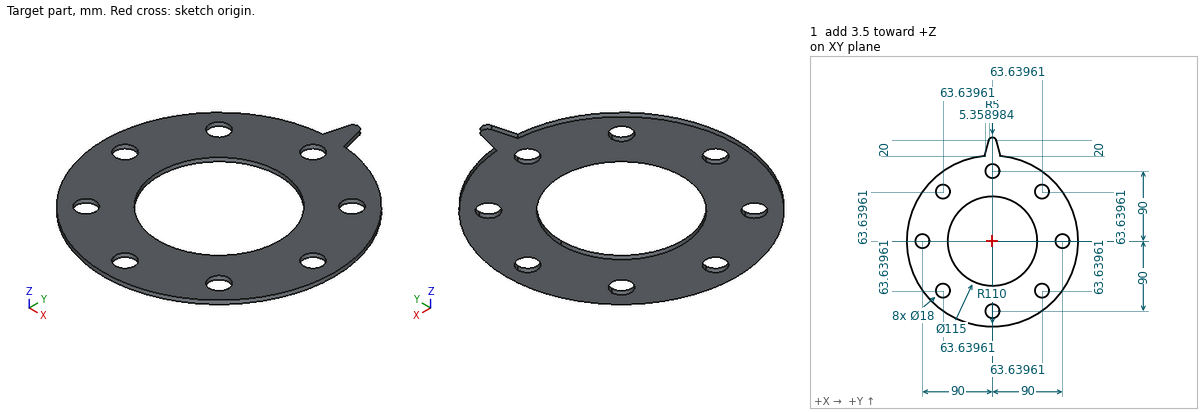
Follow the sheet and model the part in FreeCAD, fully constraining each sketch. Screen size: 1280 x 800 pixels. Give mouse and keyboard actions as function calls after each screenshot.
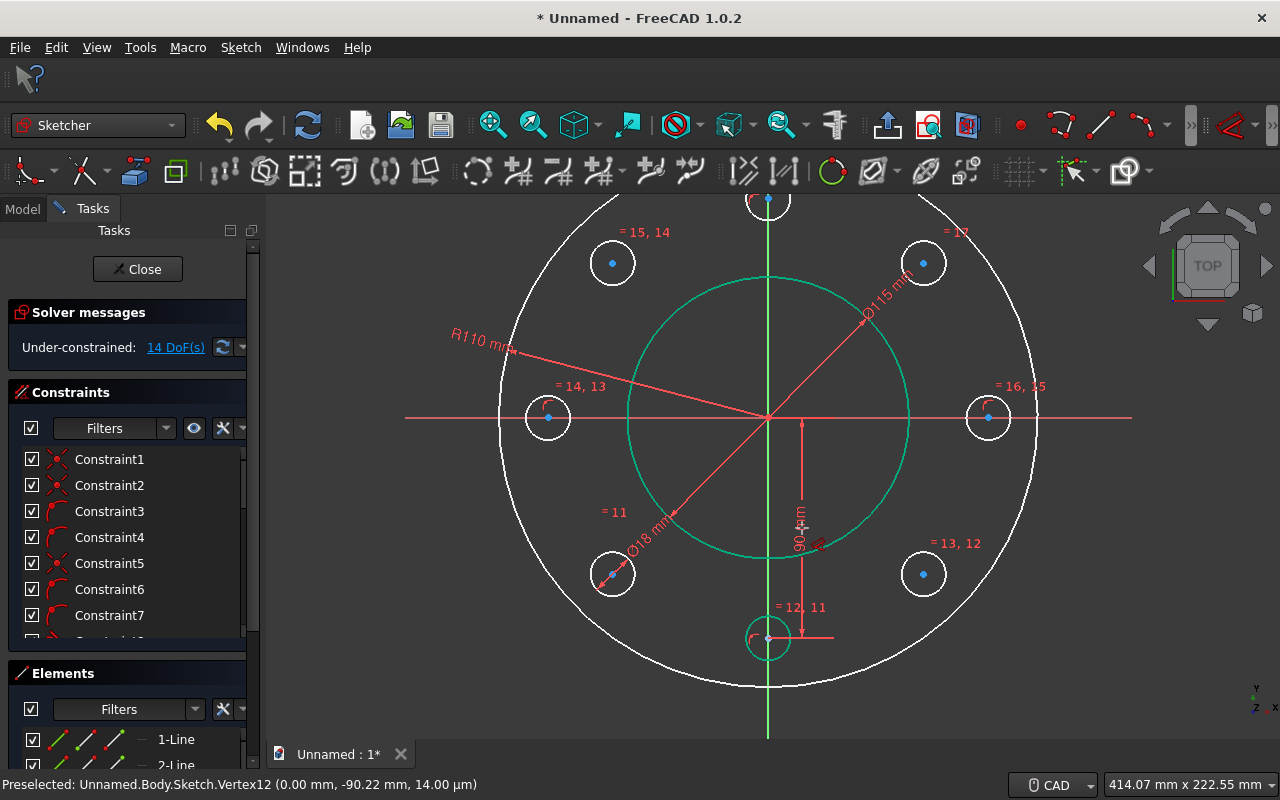
click(548, 418)
click(658, 452)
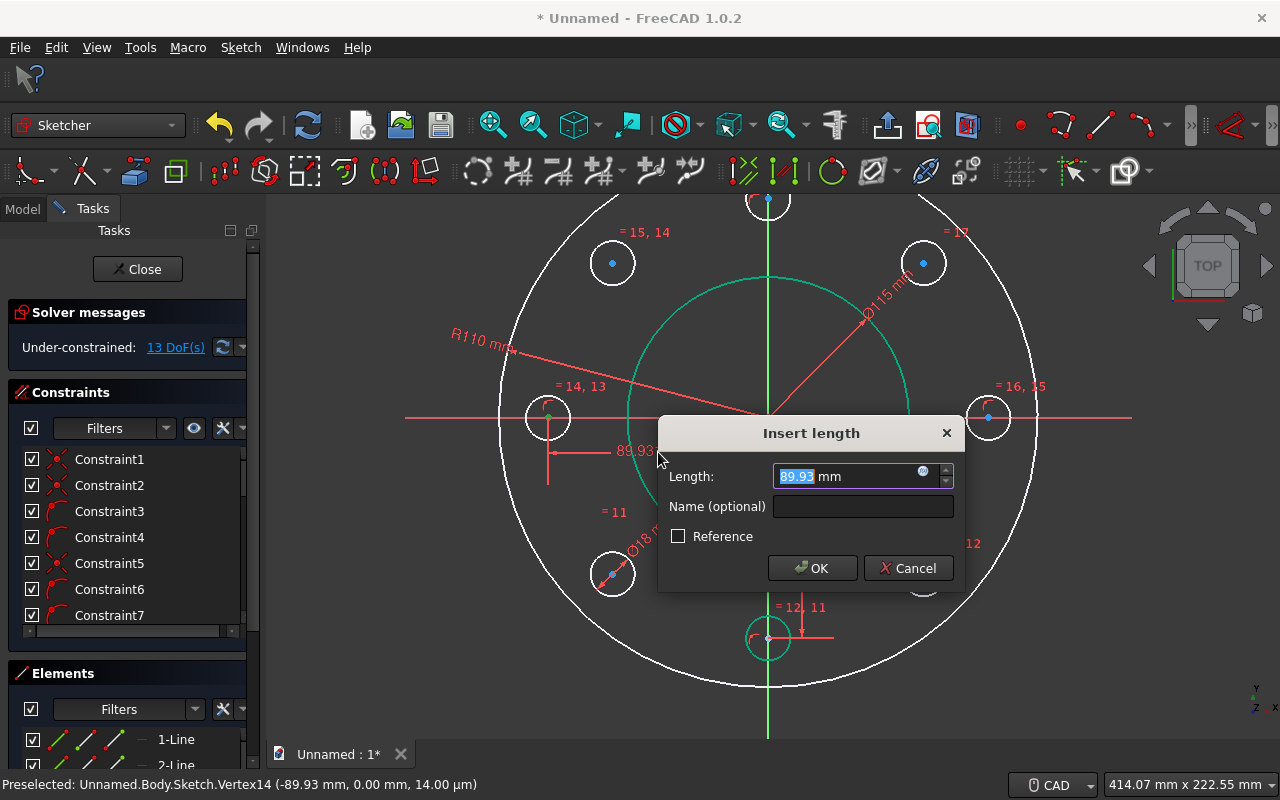
text(90)
key(Return)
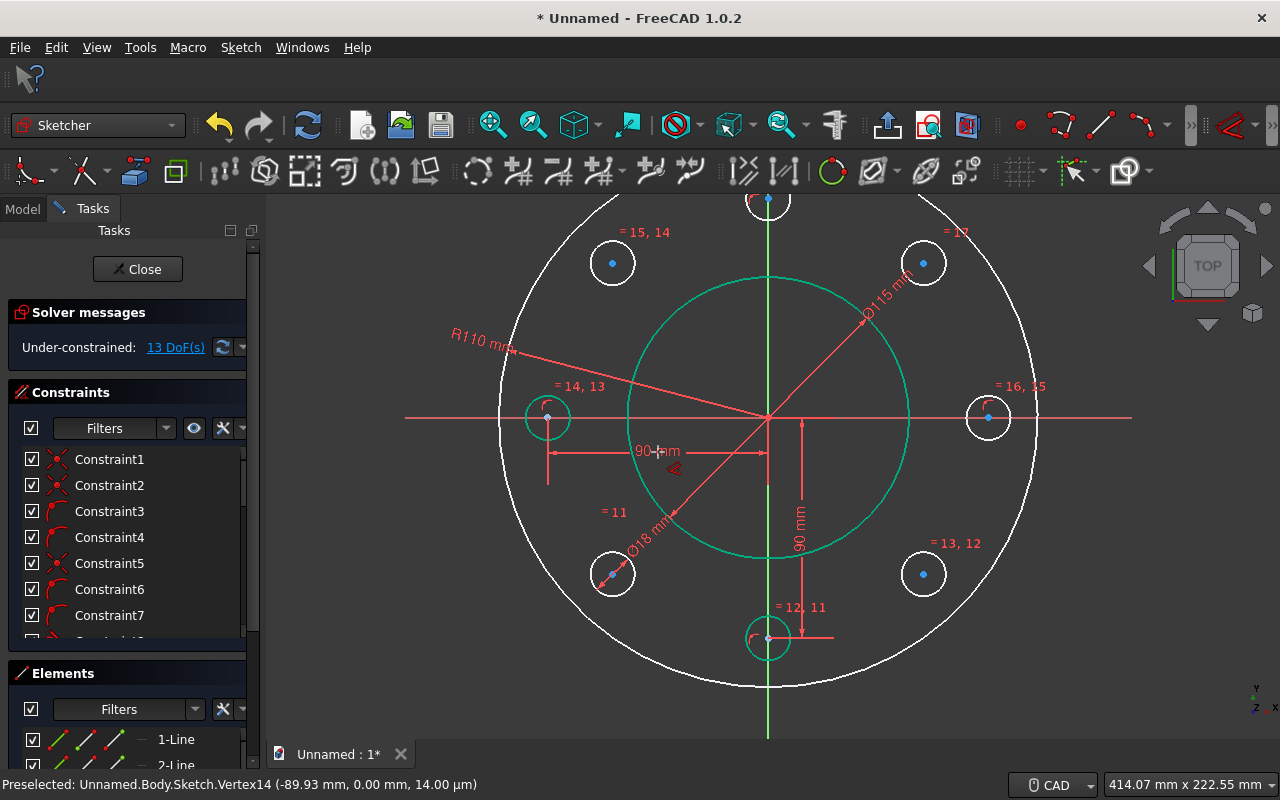
click(988, 418)
click(878, 452)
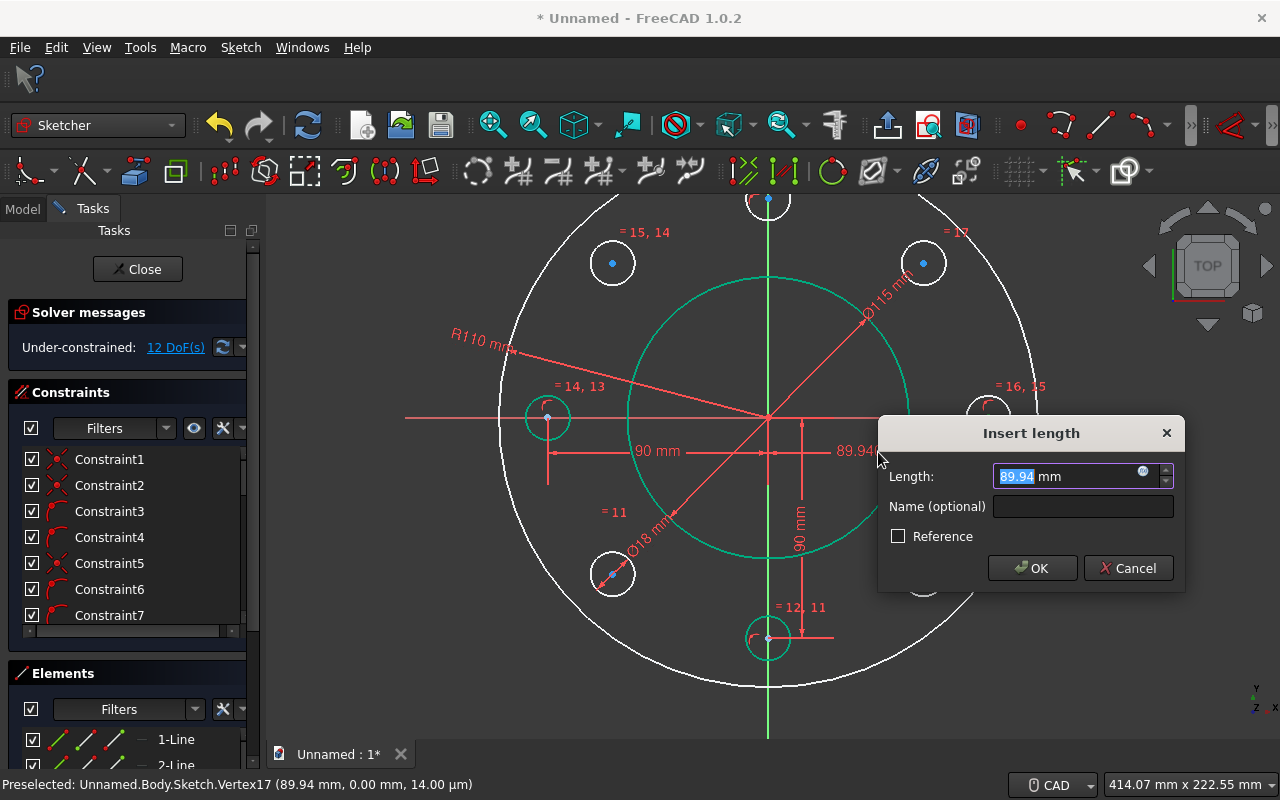
text(90)
key(Return)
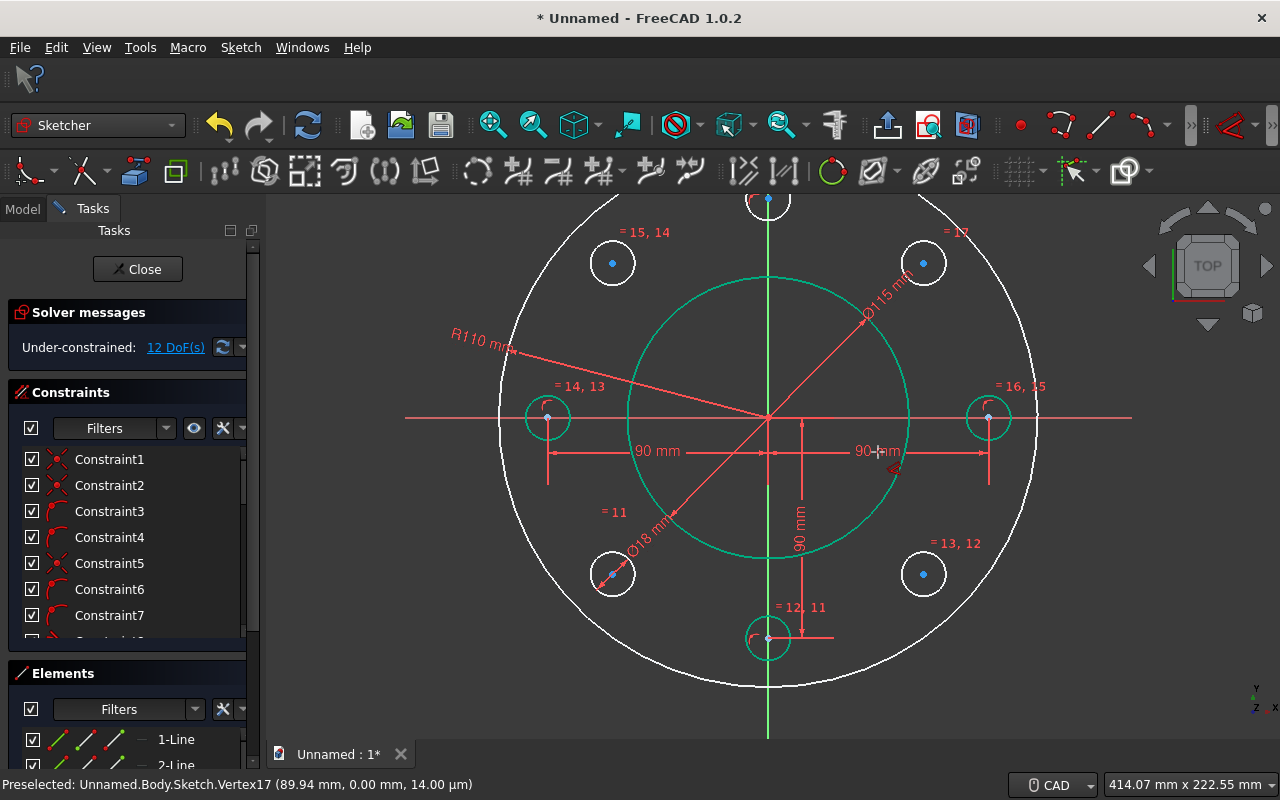
scroll(627, 560, down, 3)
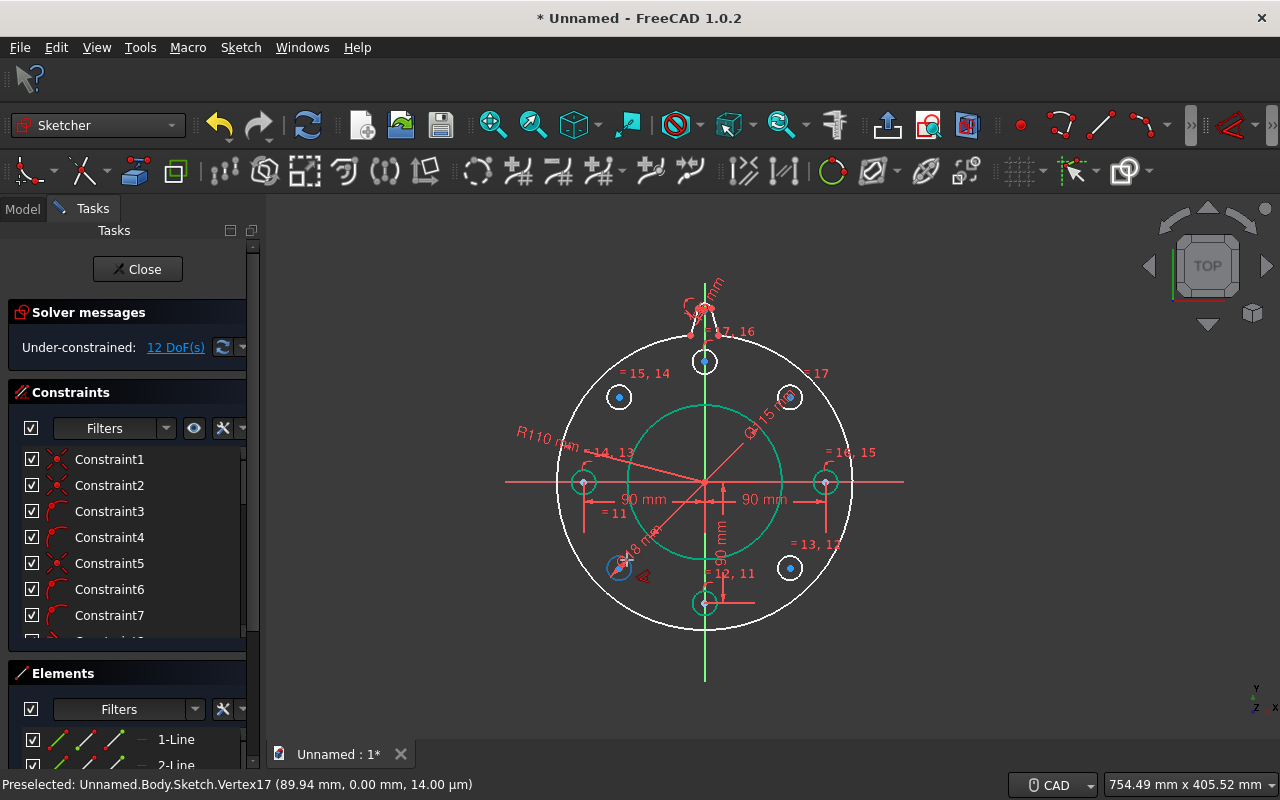
click(705, 362)
click(739, 394)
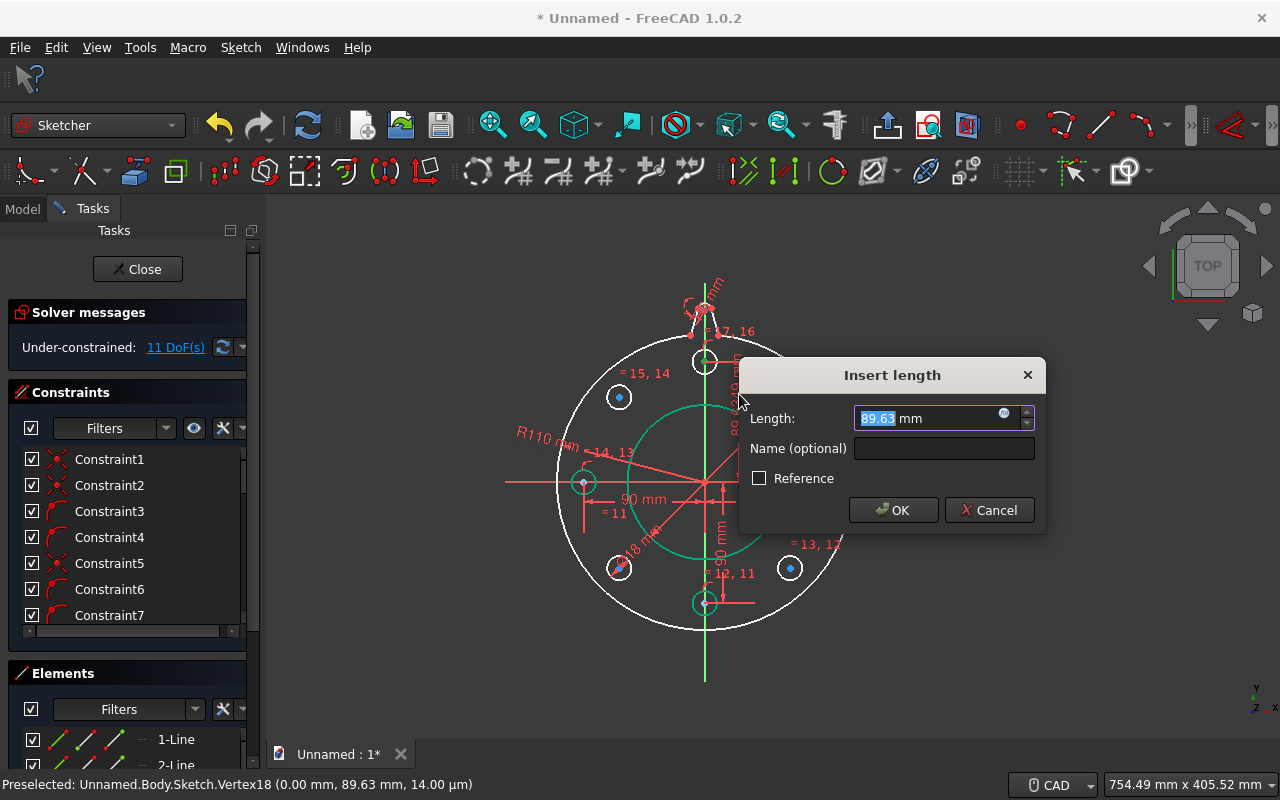
text(90)
key(Return)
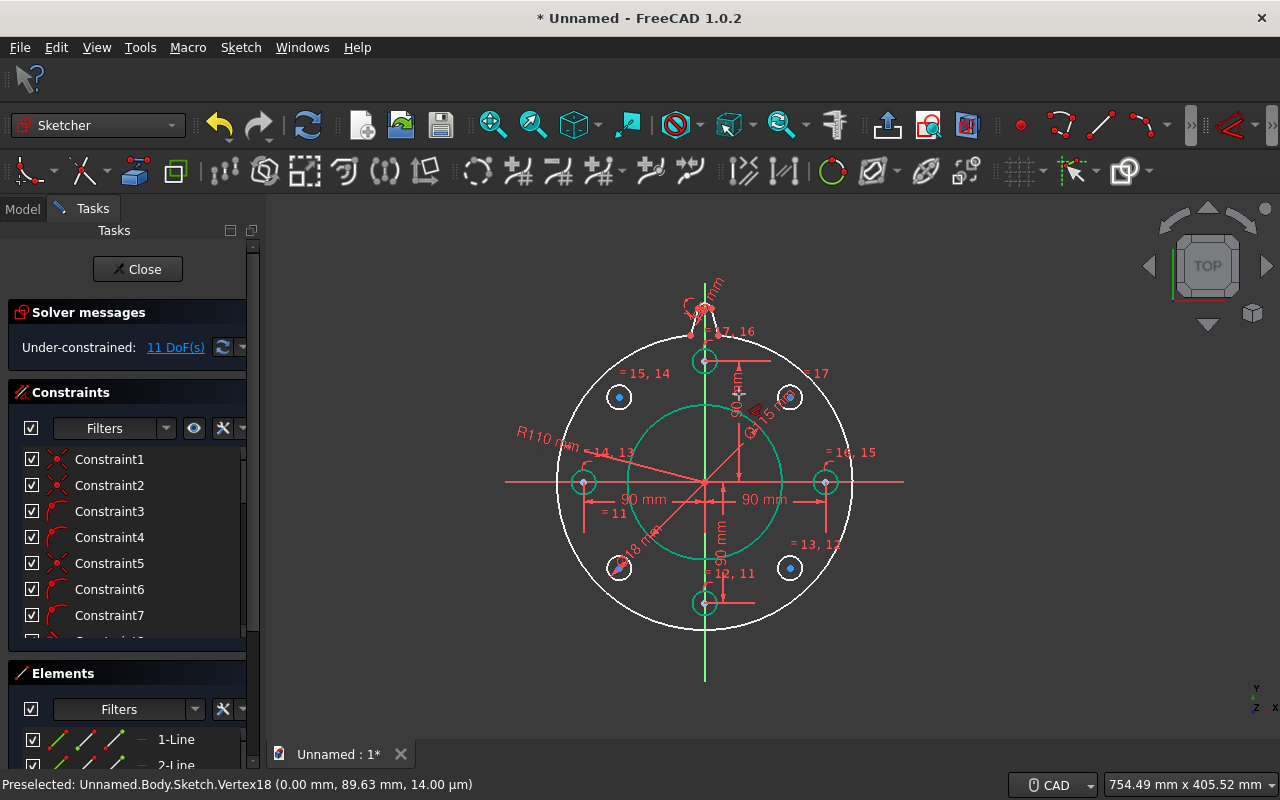
scroll(695, 319, up, 2)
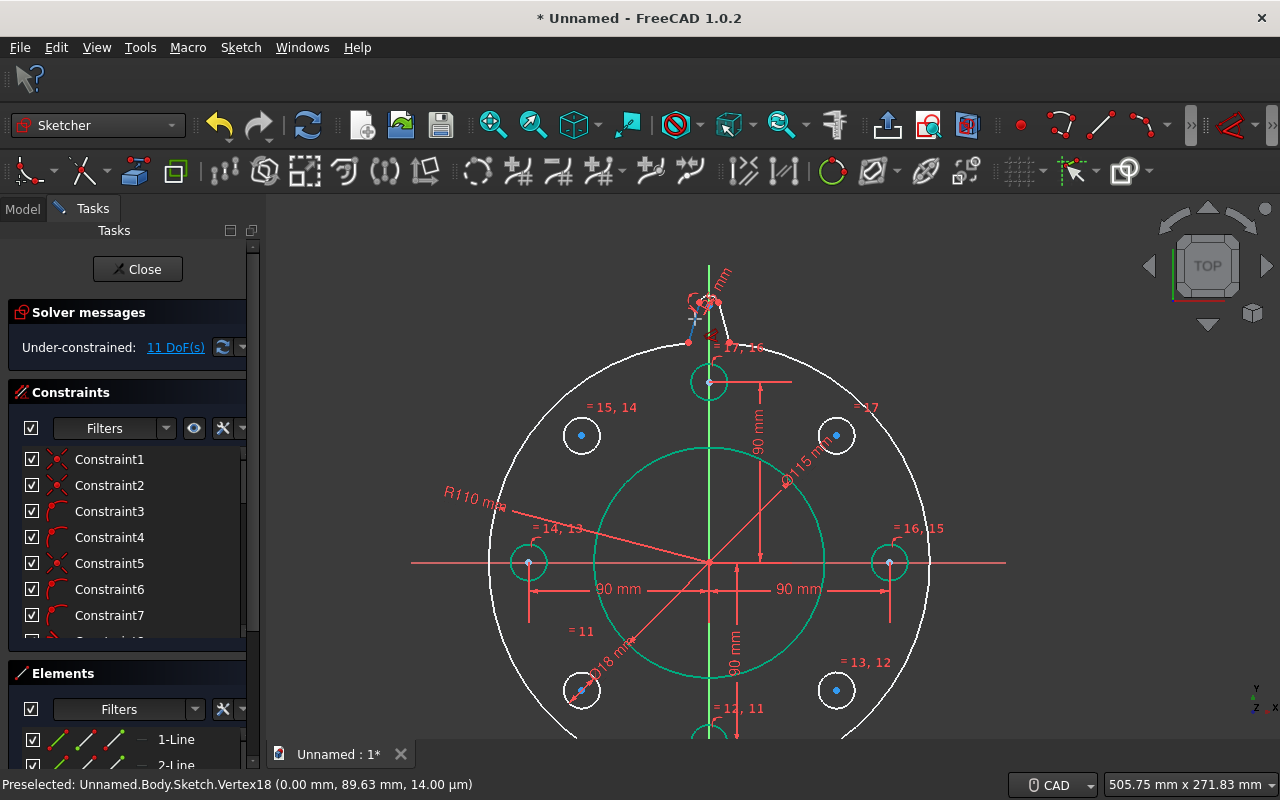
click(695, 319)
click(655, 323)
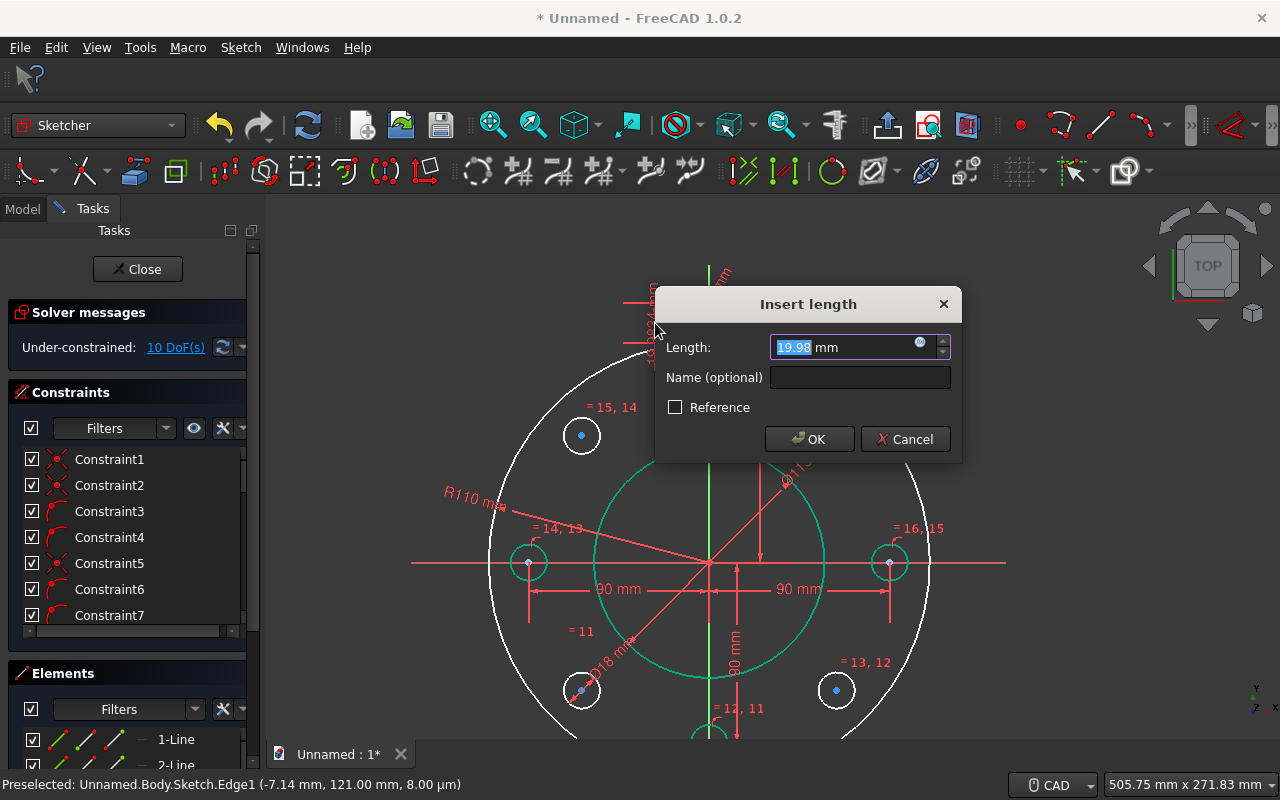
text(20)
key(Return)